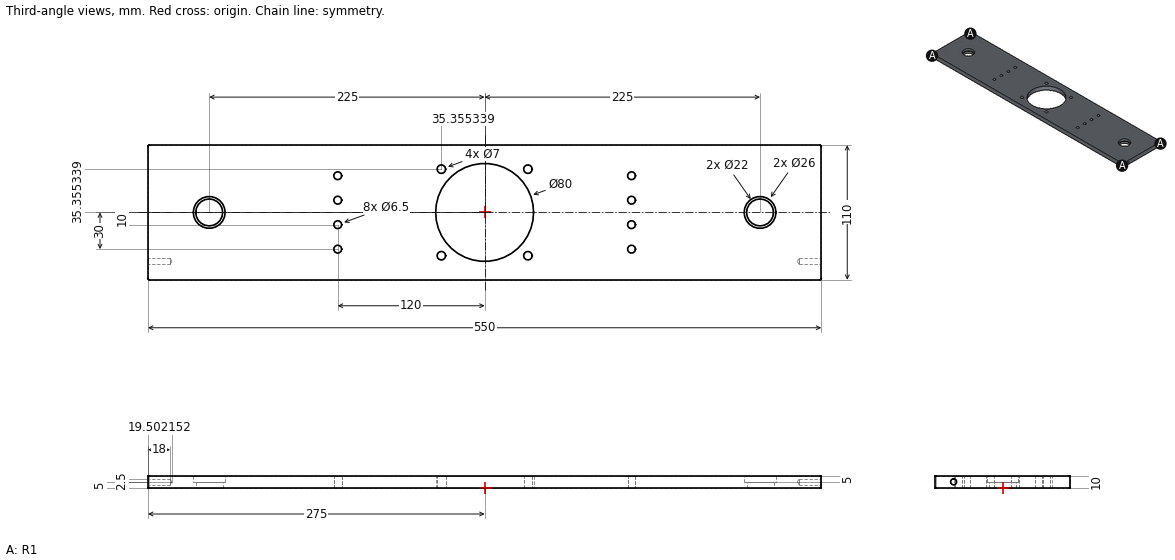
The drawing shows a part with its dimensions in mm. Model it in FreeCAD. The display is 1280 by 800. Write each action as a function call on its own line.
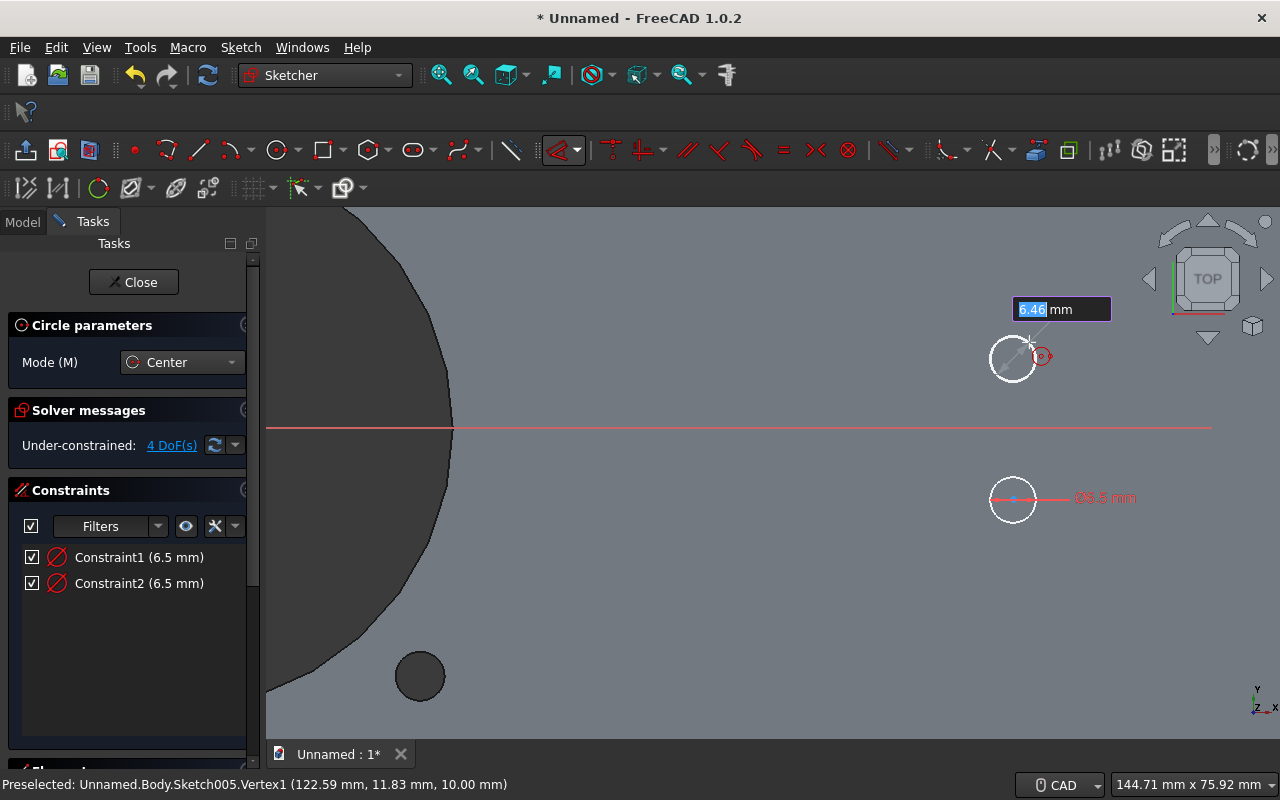
text(6.5)
key(Return)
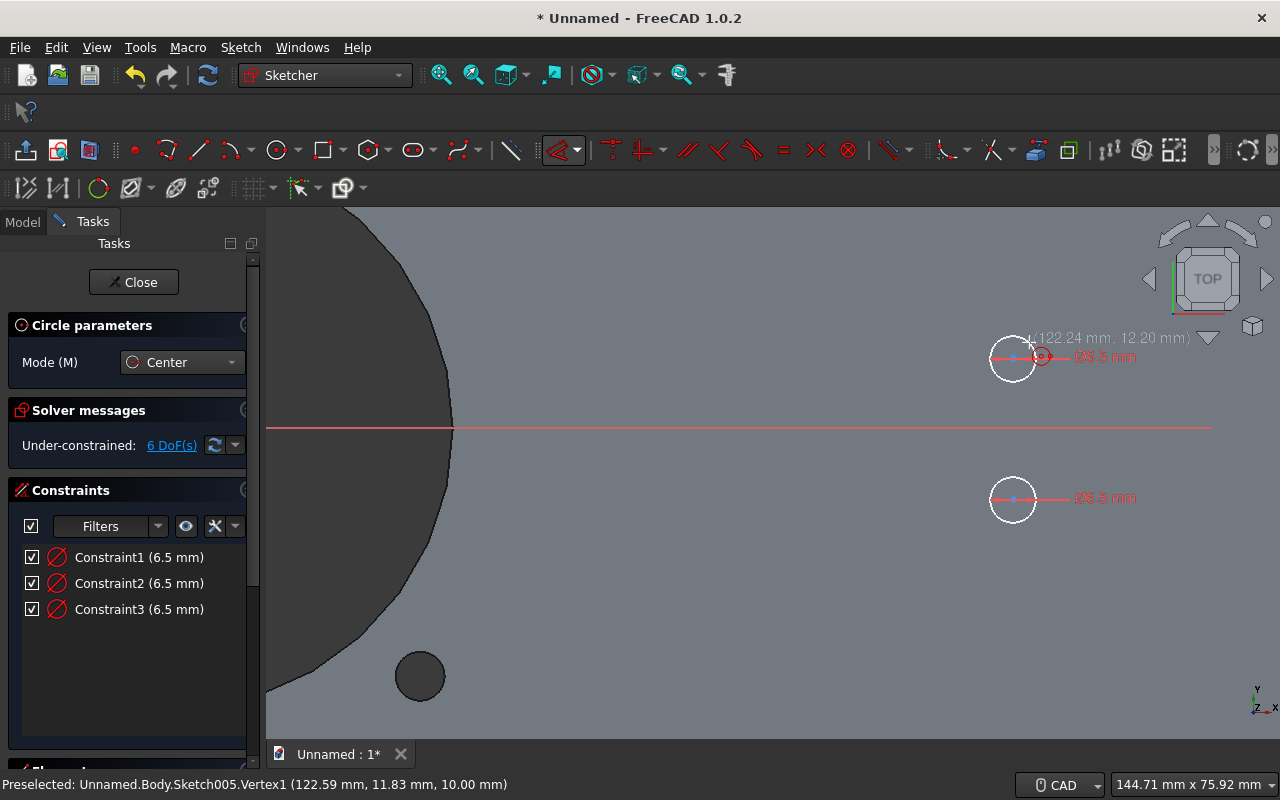
scroll(1014, 499, down, 5)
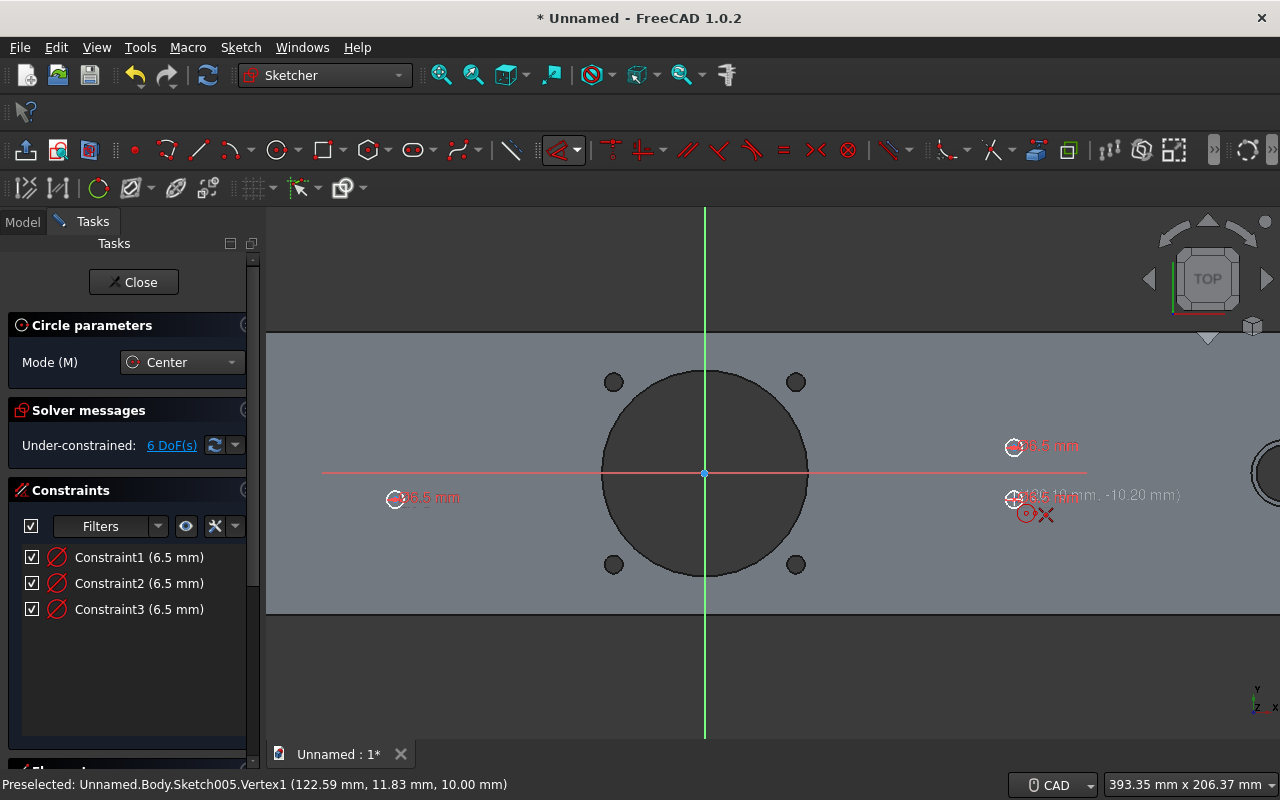
scroll(396, 448, up, 5)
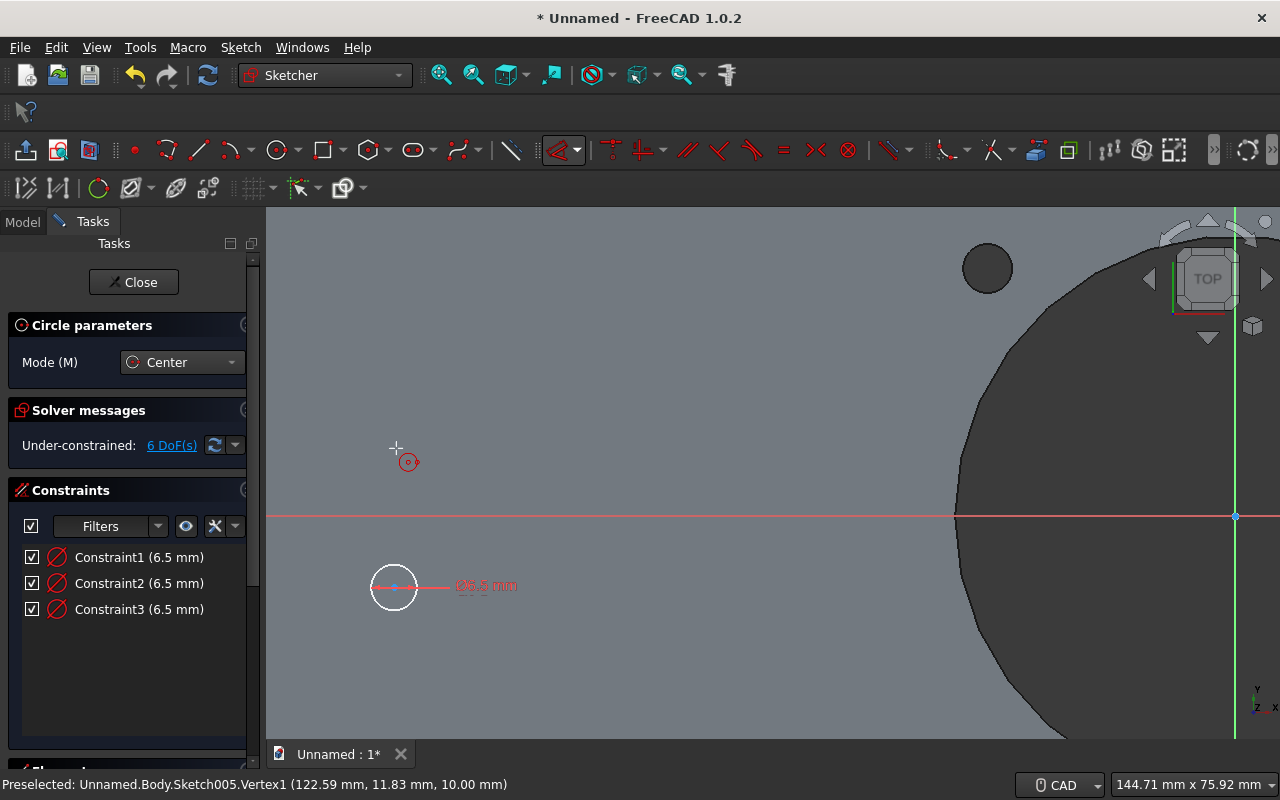
click(394, 446)
move(411, 430)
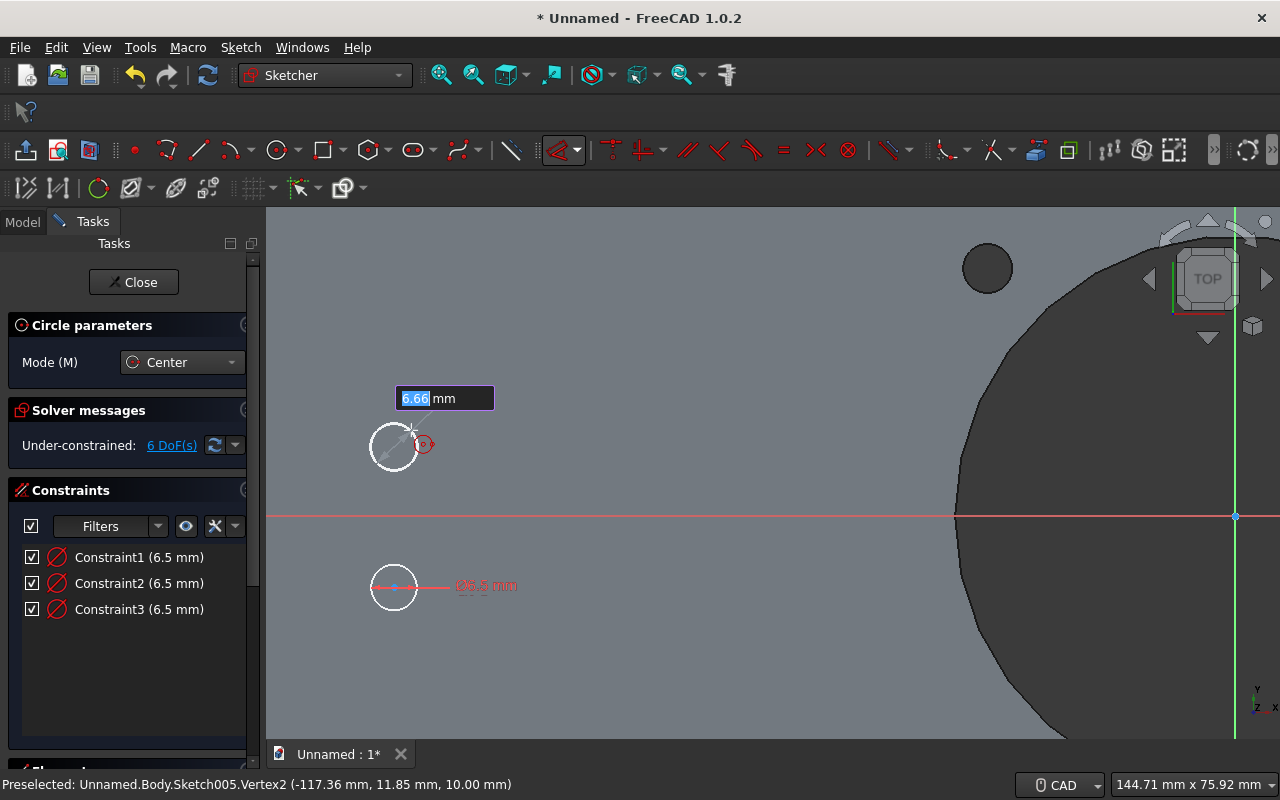
text(6.5)
key(Return)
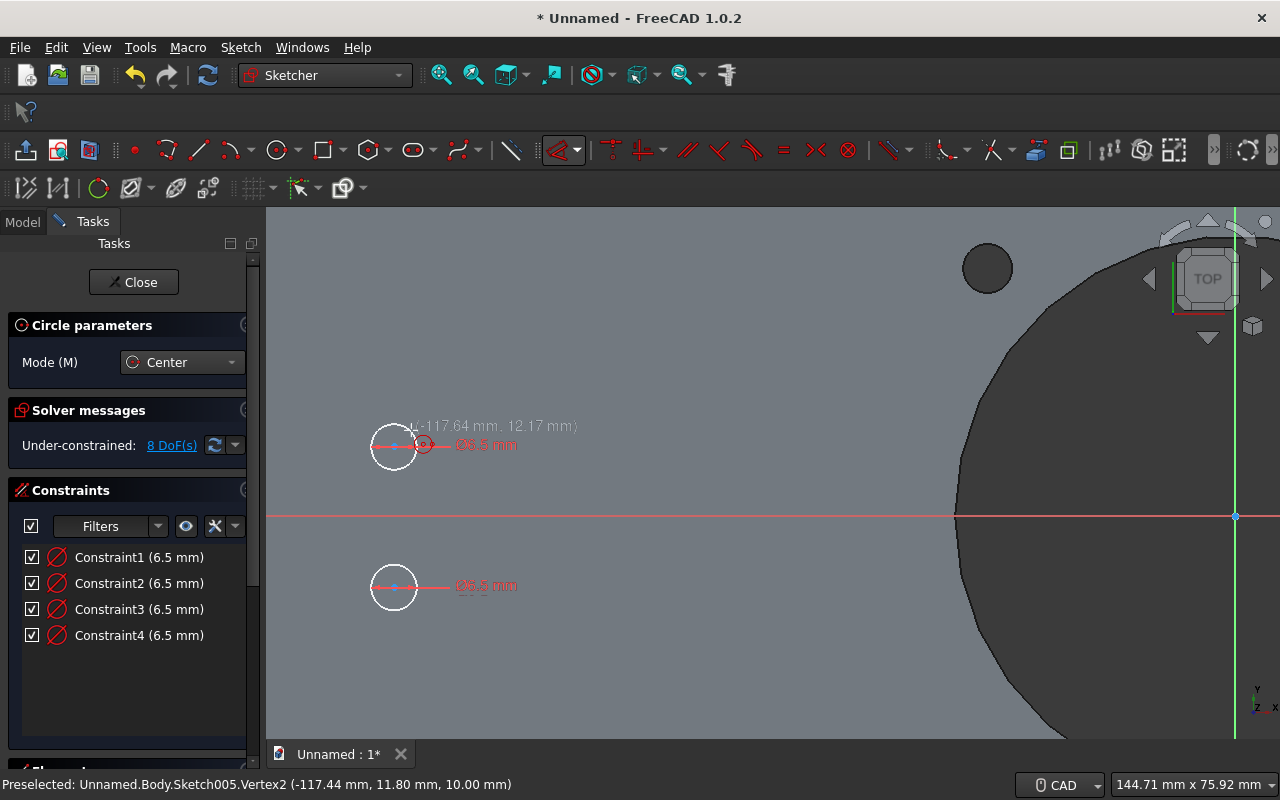
scroll(396, 448, down, 5)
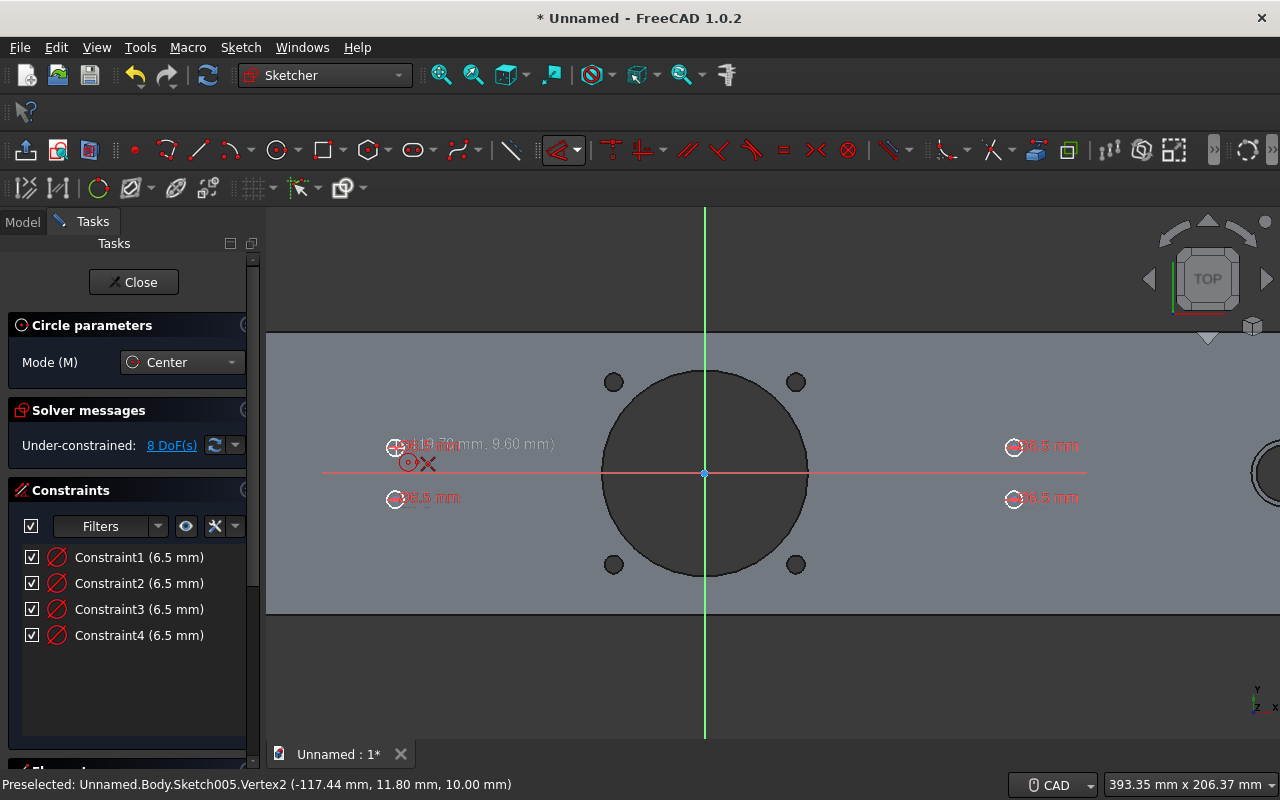
scroll(396, 551, up, 5)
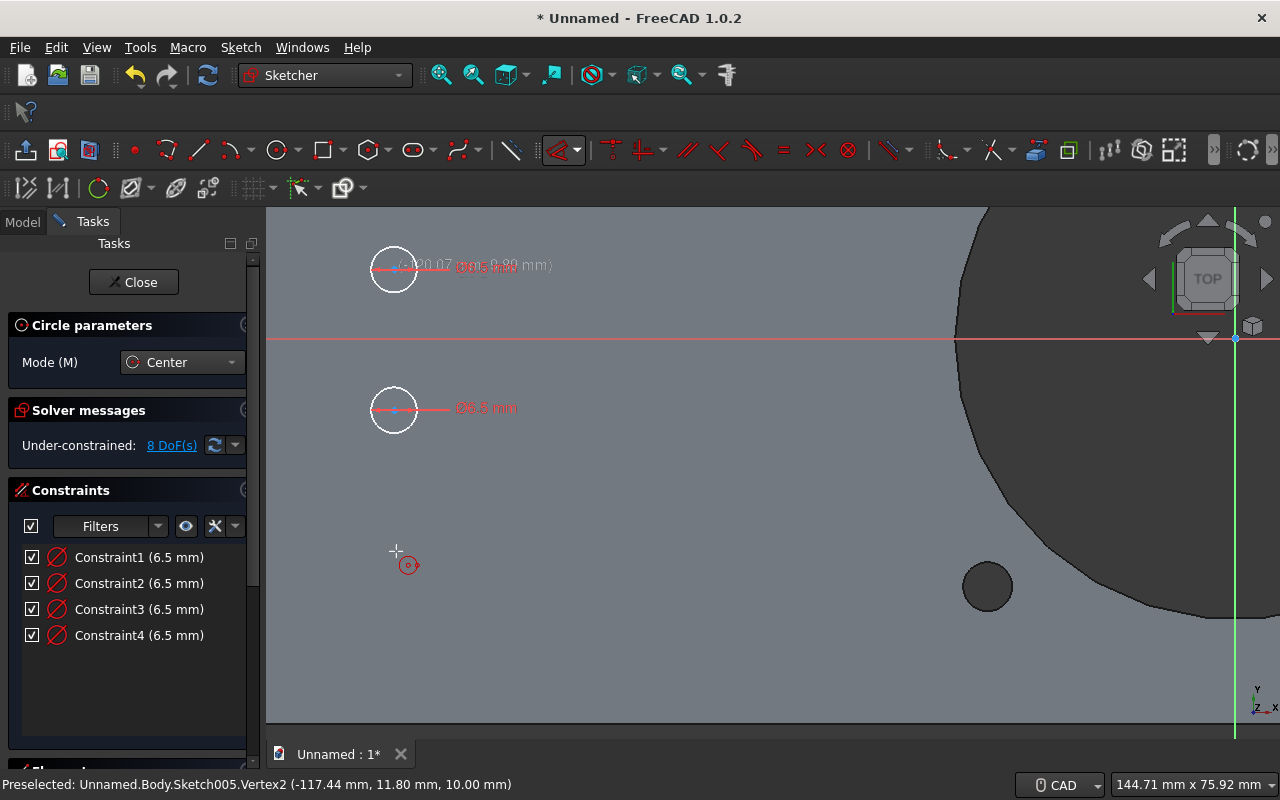
click(394, 549)
move(411, 533)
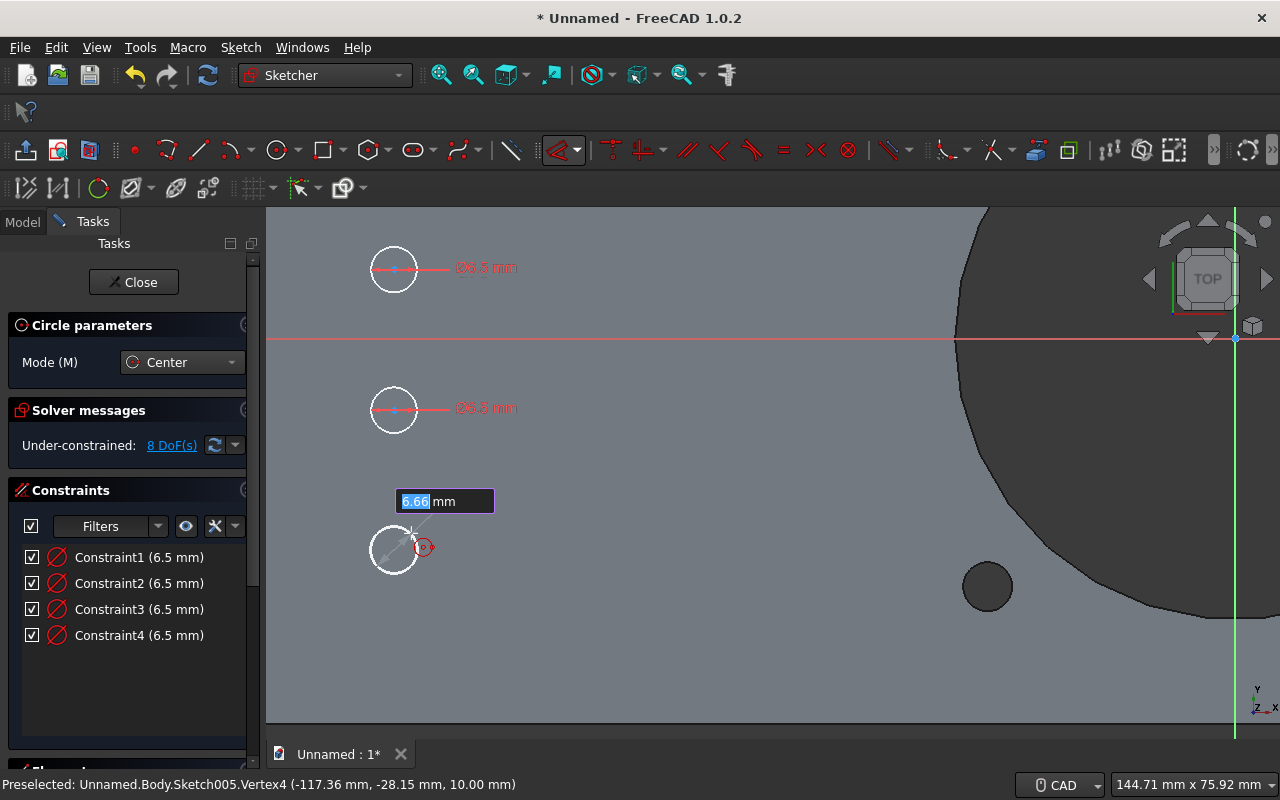
text(6.5)
key(Return)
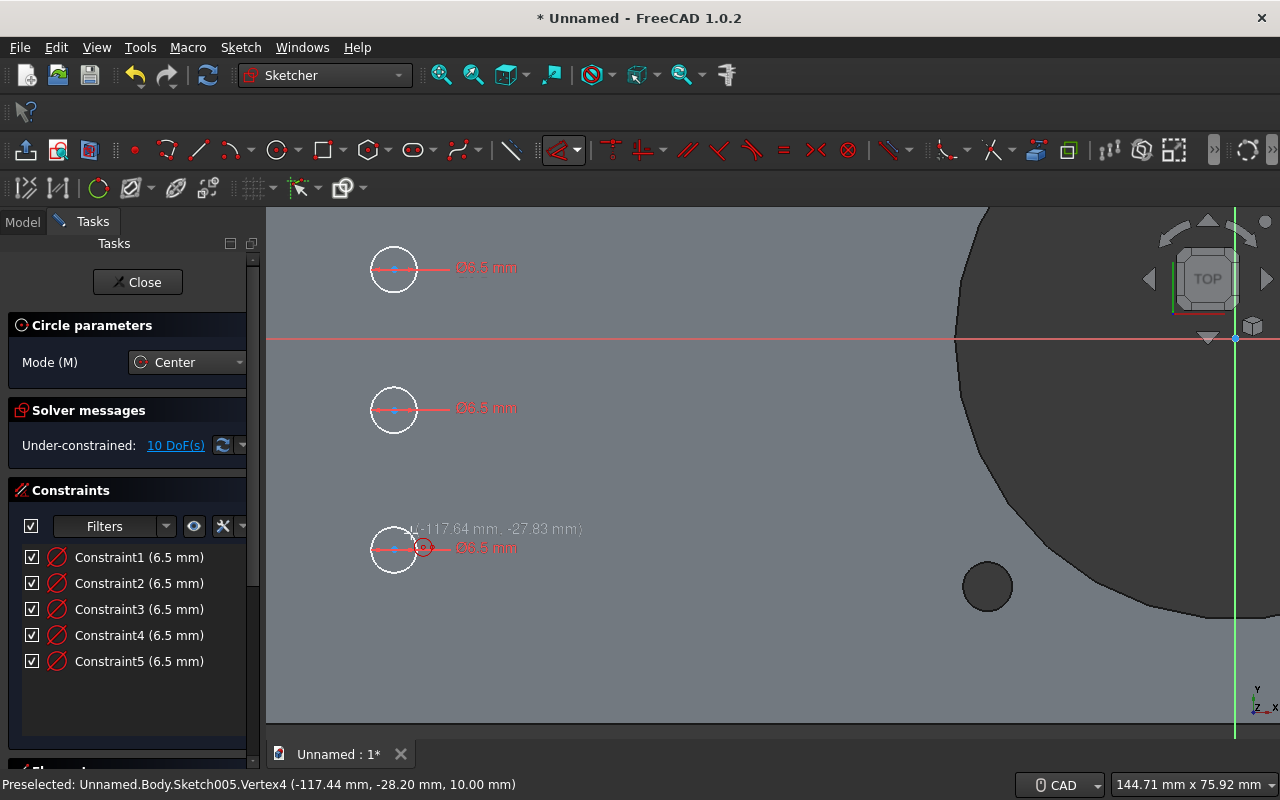
scroll(396, 551, down, 5)